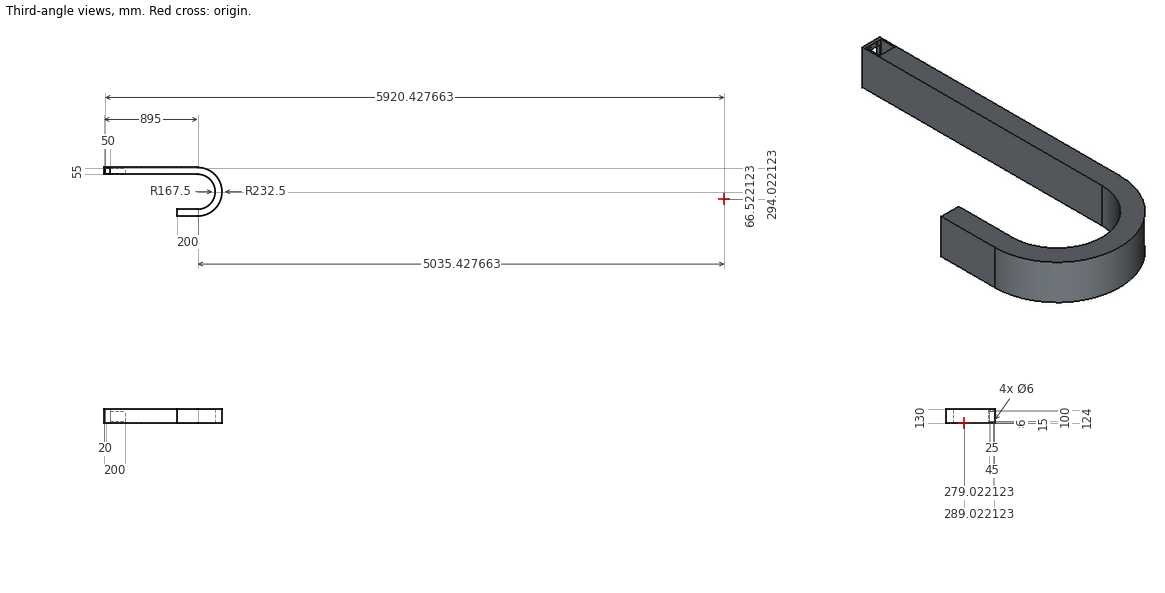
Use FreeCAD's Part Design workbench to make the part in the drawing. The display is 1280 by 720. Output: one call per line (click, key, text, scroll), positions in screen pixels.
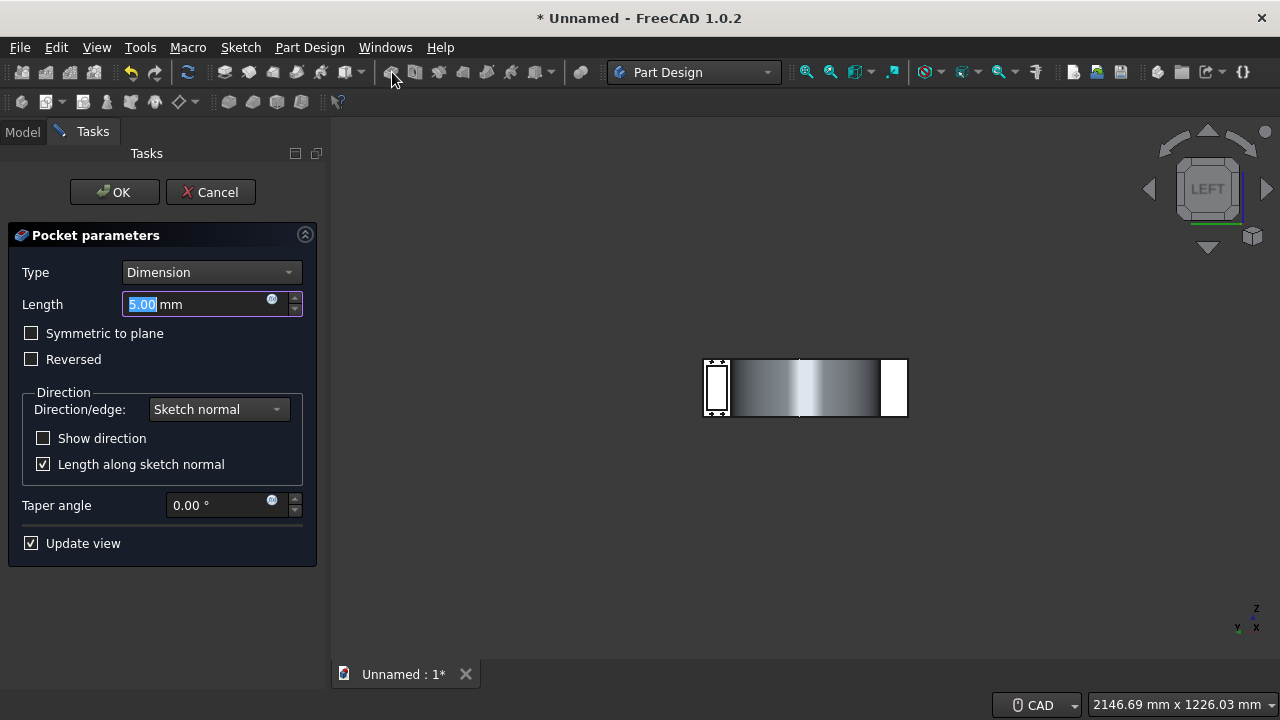
text(200)
key(Tab)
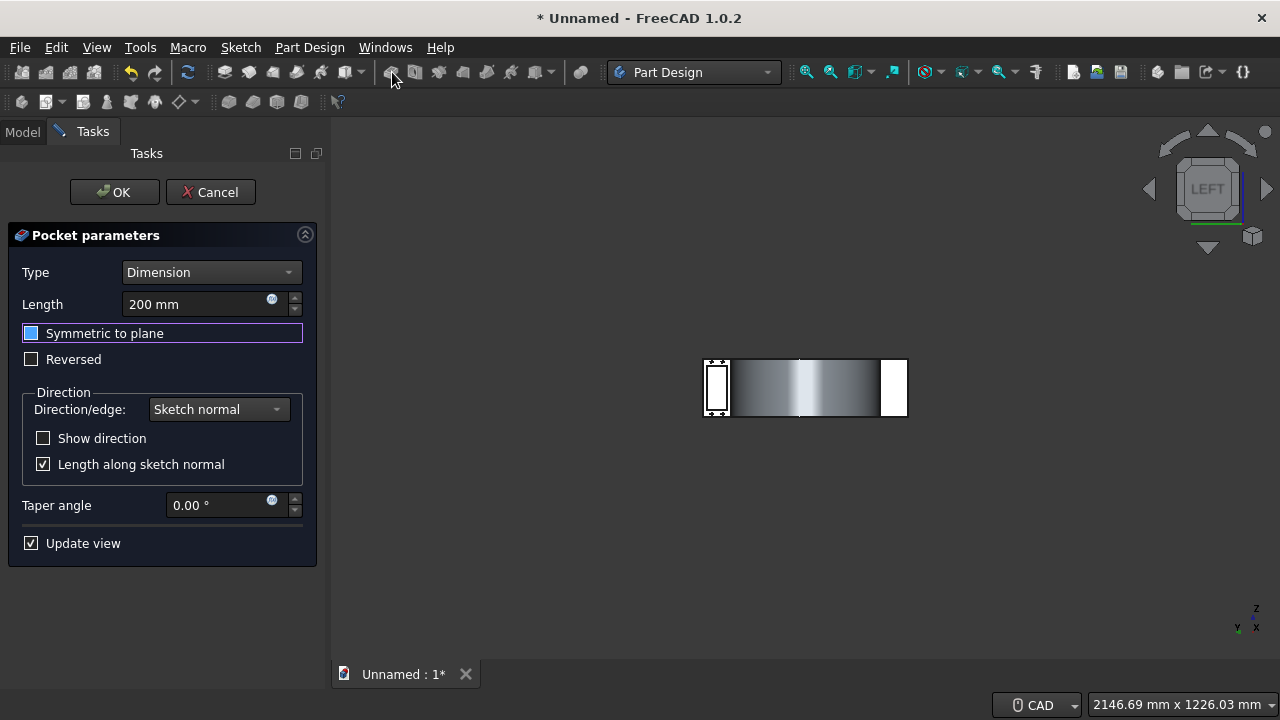
click(115, 192)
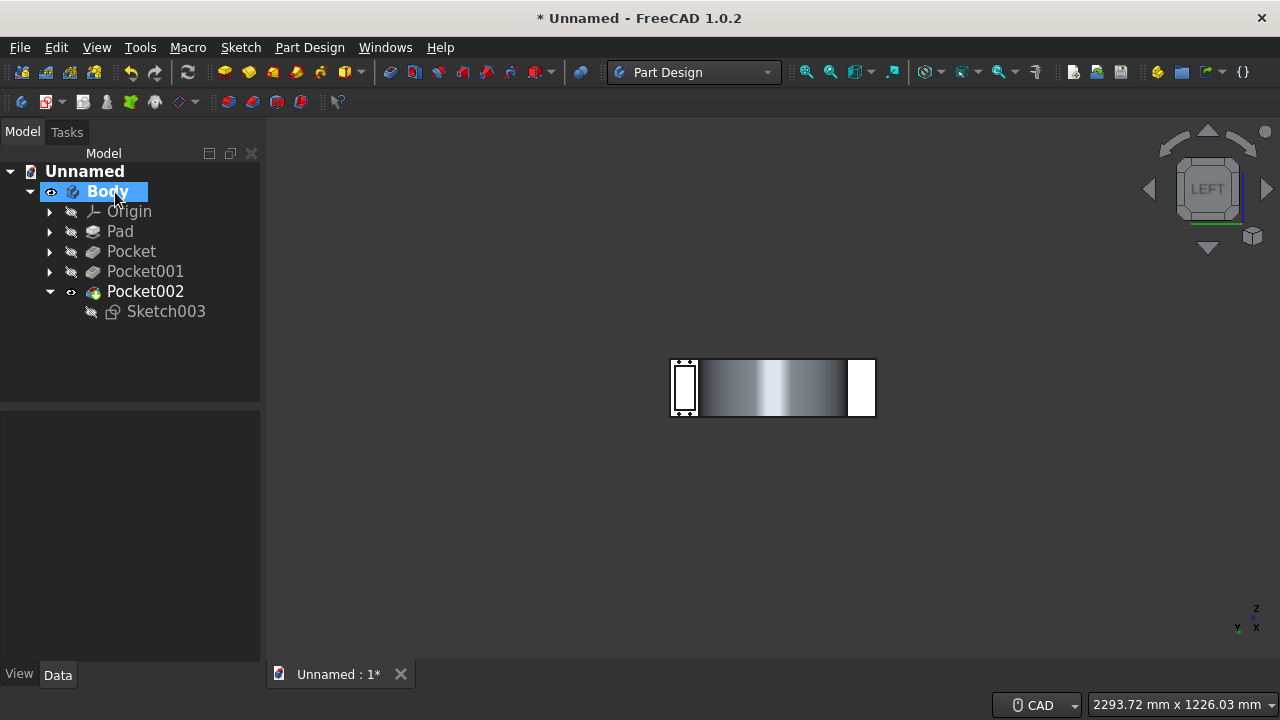
key(0)